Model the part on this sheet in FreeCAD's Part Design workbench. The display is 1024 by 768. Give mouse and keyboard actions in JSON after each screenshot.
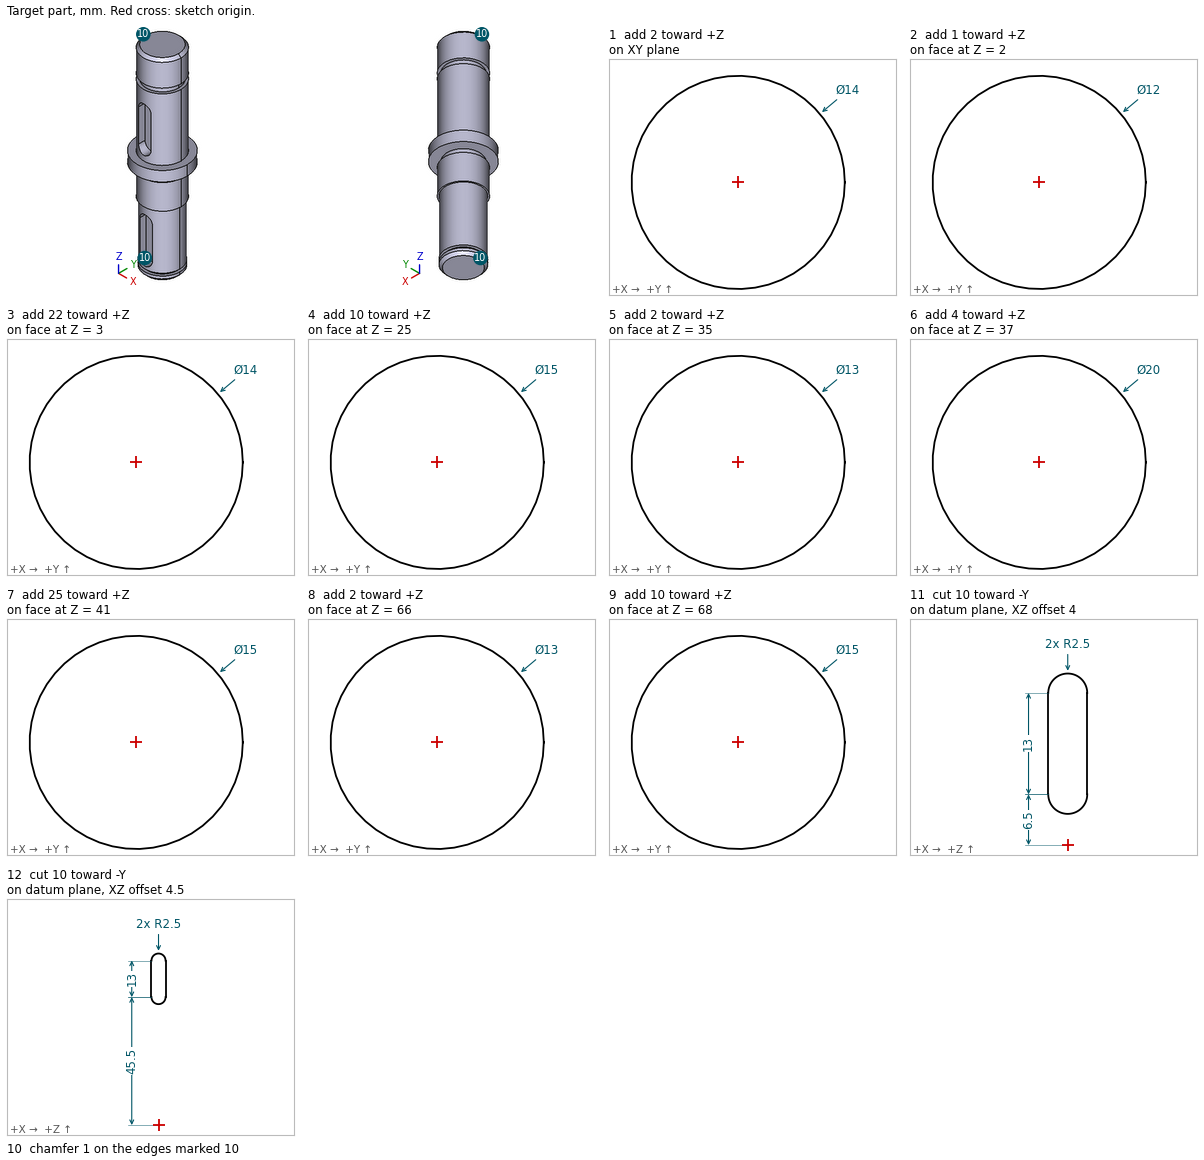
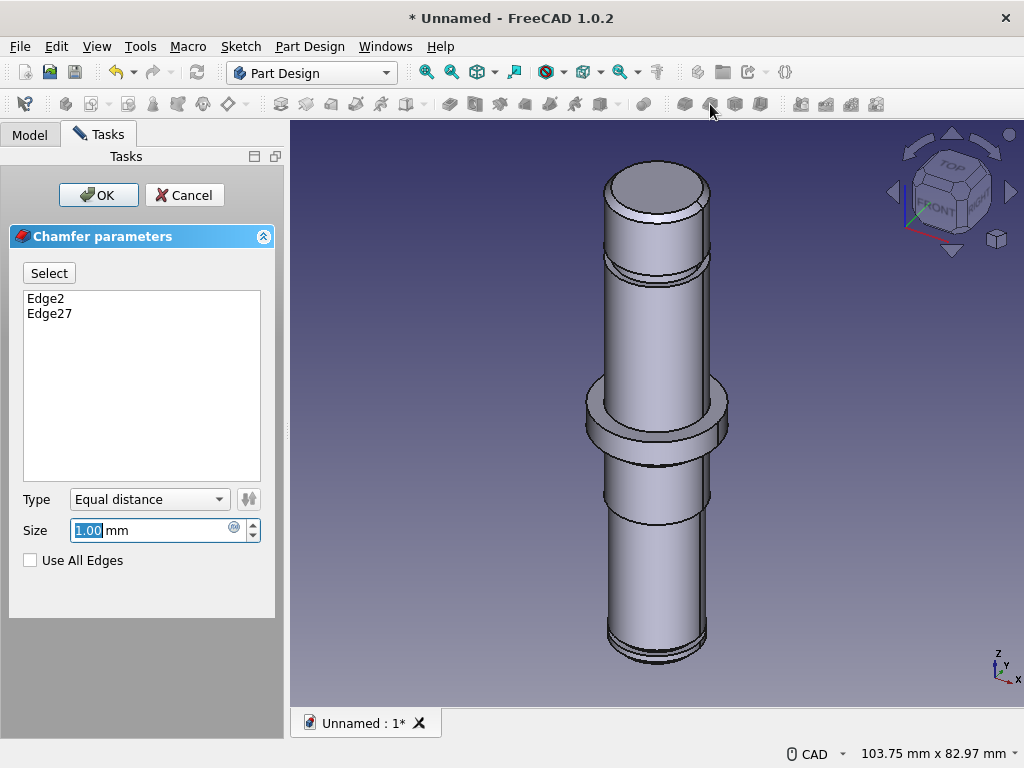
{"action": "type", "text": "1"}
{"action": "key", "text": "Tab"}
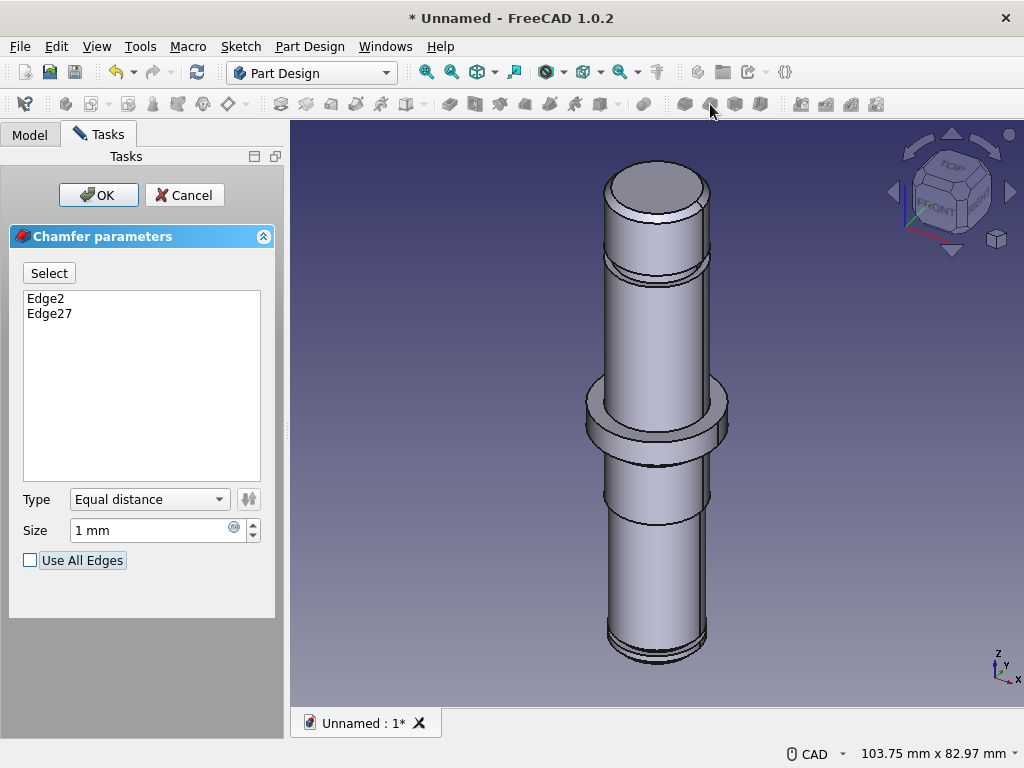
{"action": "left_click", "coordinate": [99, 195]}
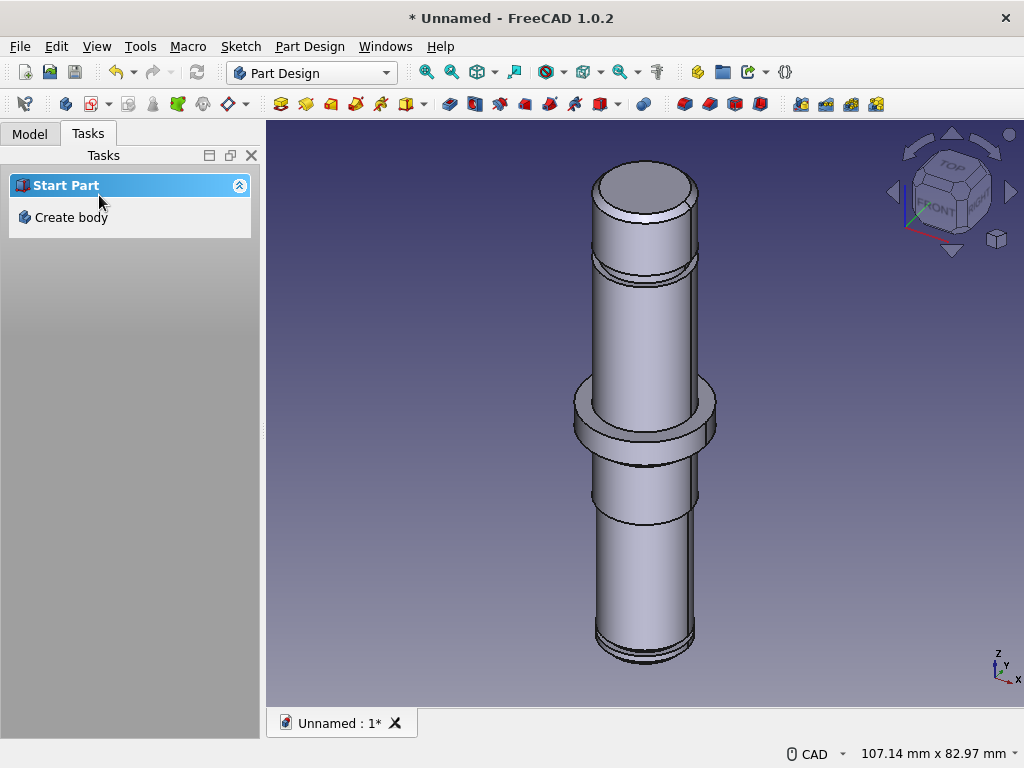
{"action": "left_click", "coordinate": [30, 134]}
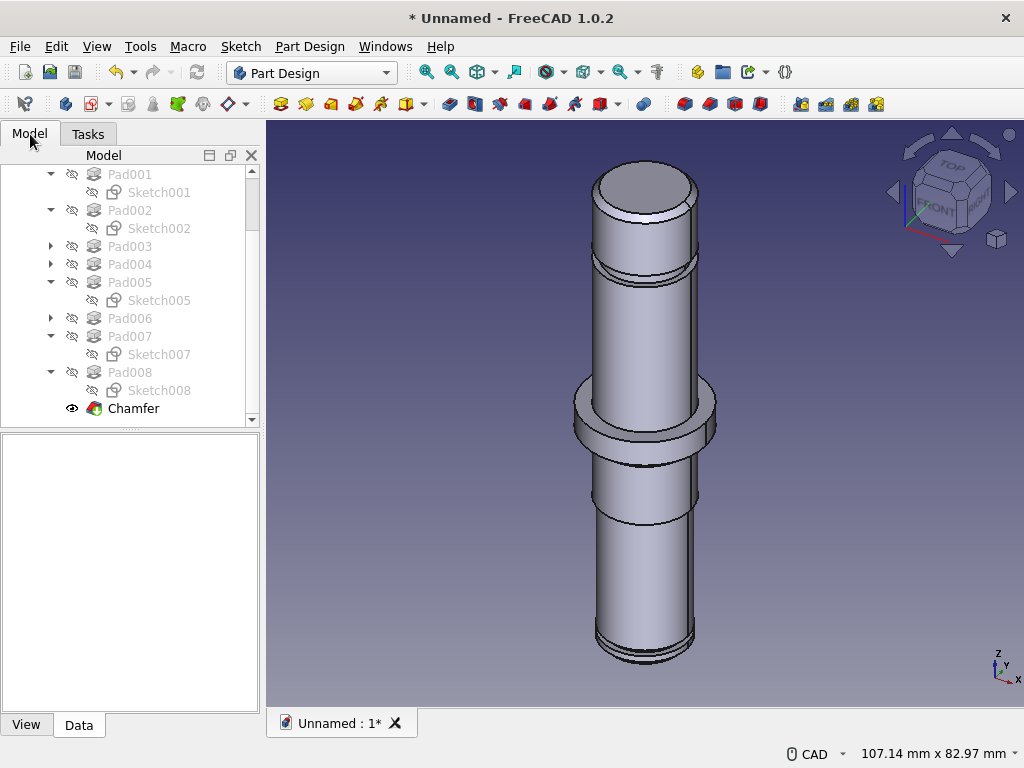
{"action": "scroll", "coordinate": [141, 296], "scroll_direction": "down", "scroll_amount": 3}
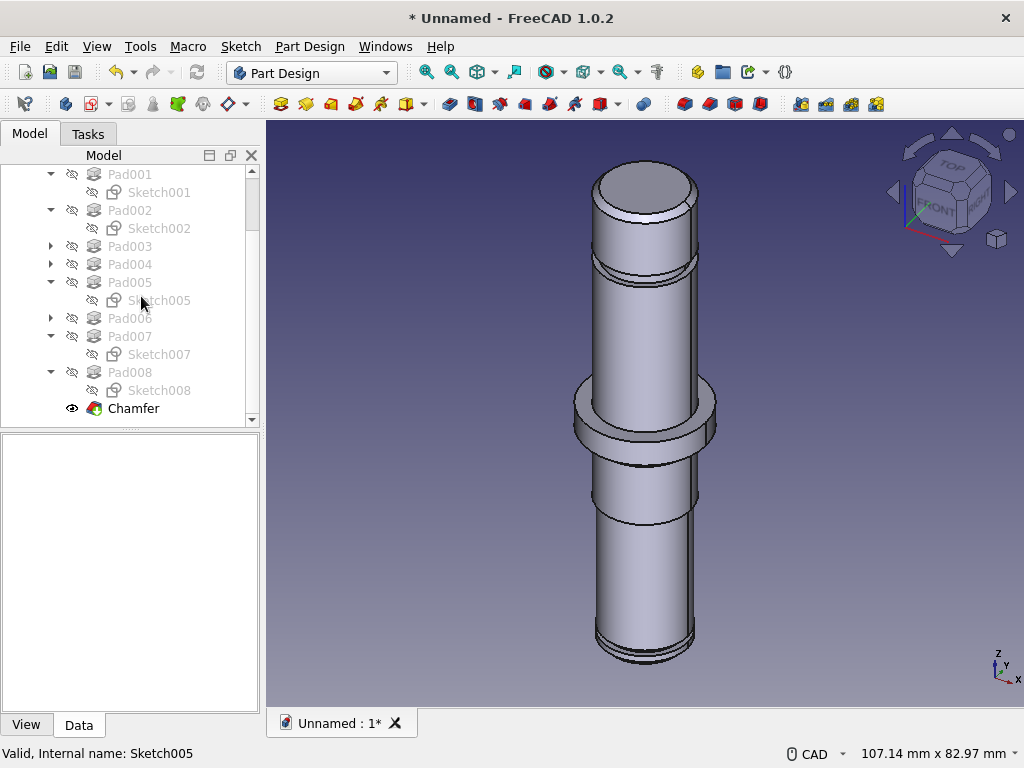
{"action": "scroll", "coordinate": [141, 296], "scroll_direction": "up", "scroll_amount": 15}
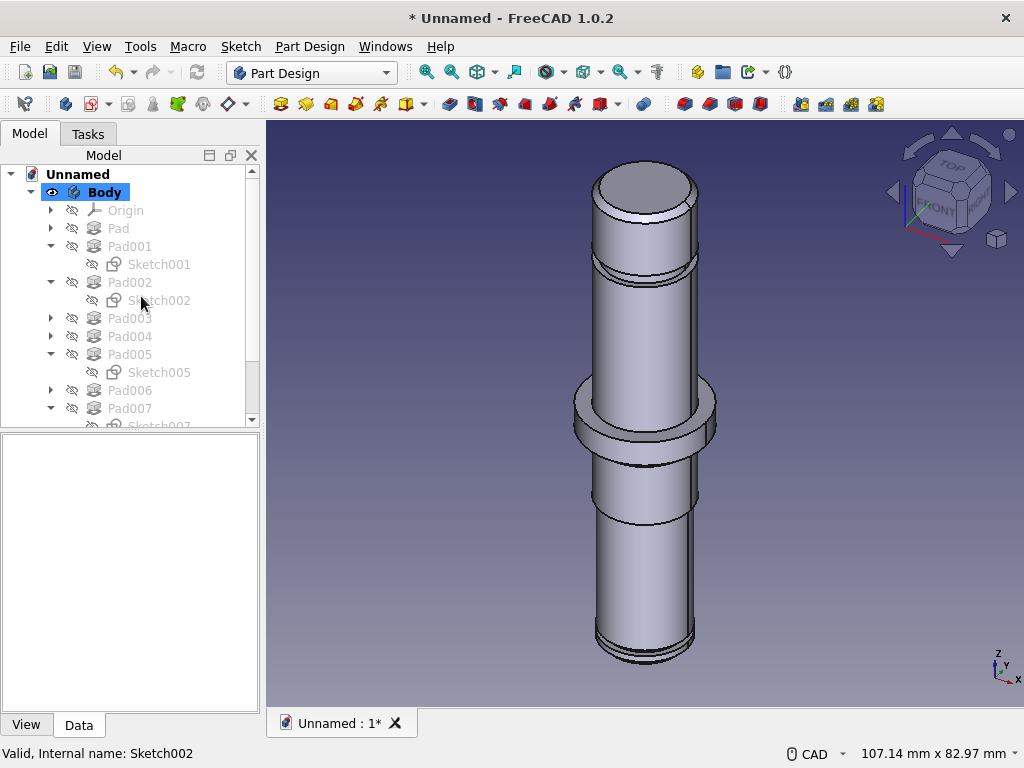
{"action": "left_click", "coordinate": [51, 210]}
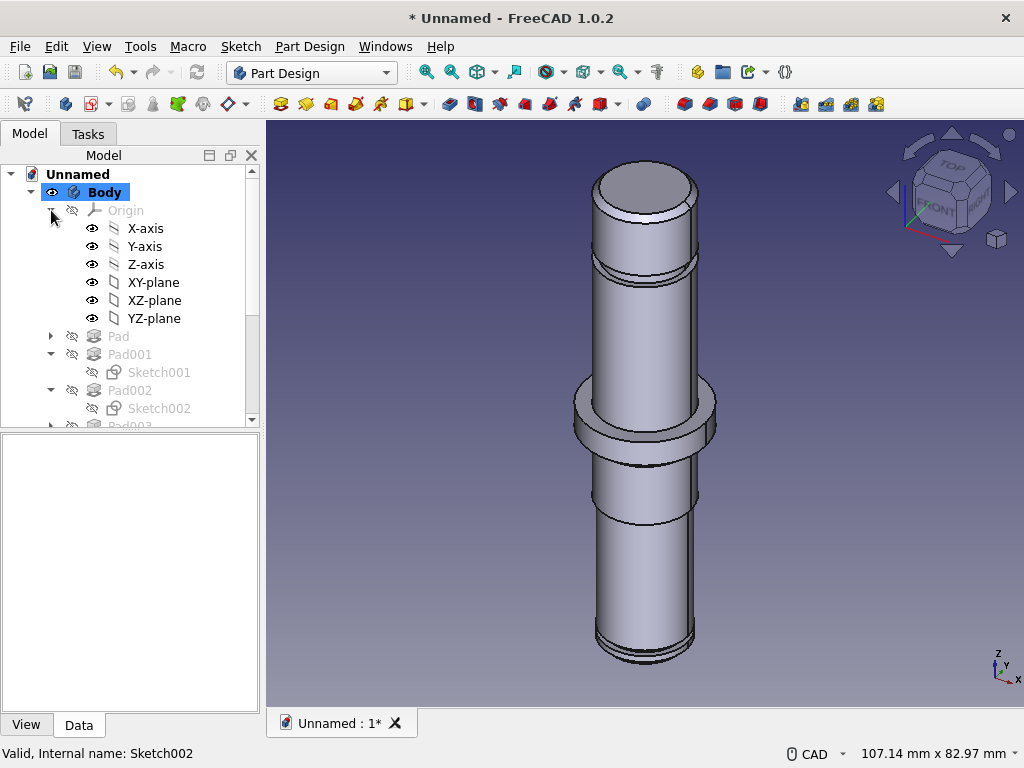
{"action": "left_click", "coordinate": [137, 300]}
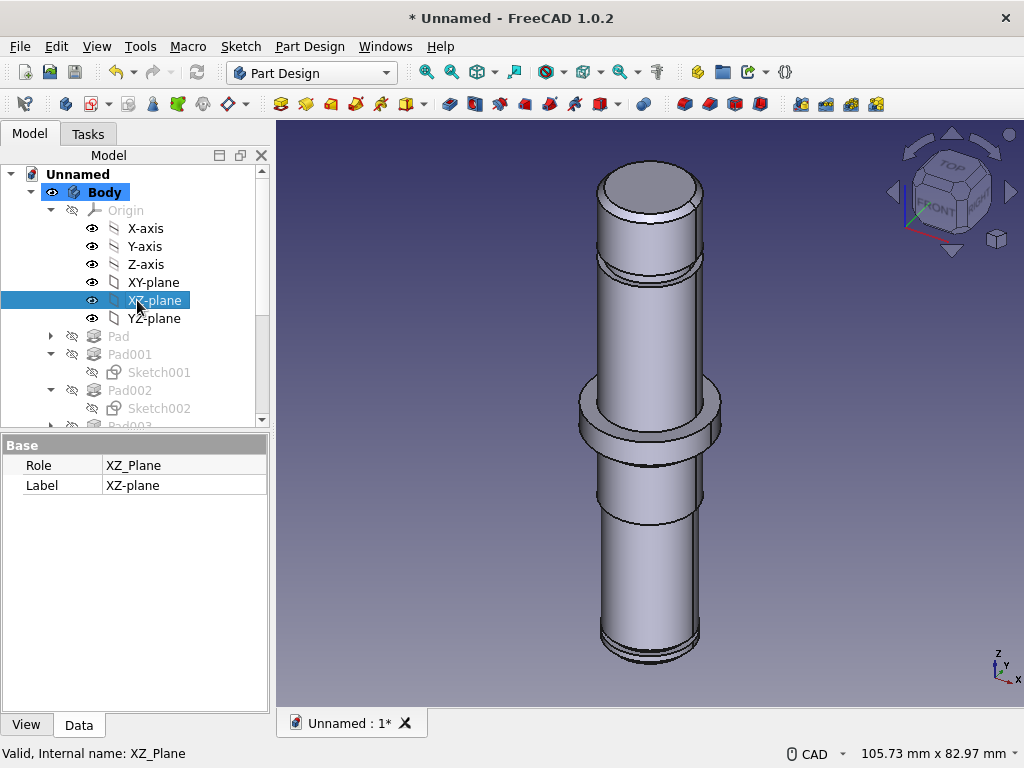
{"action": "left_click", "coordinate": [228, 104]}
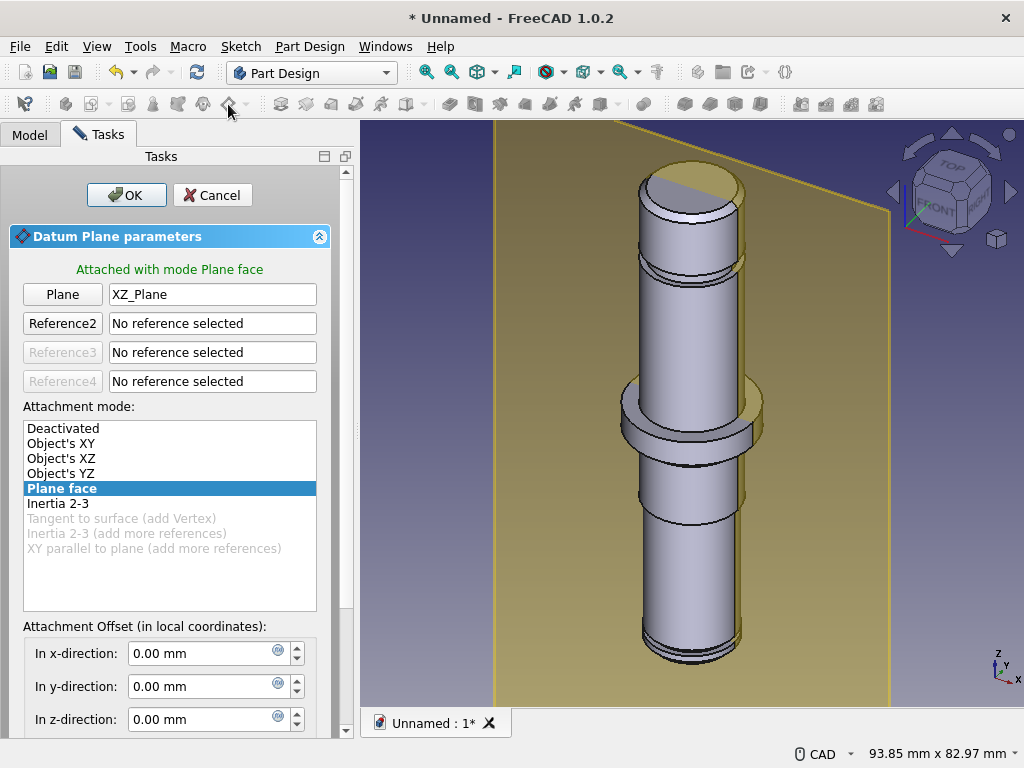
{"action": "triple_click", "coordinate": [210, 720]}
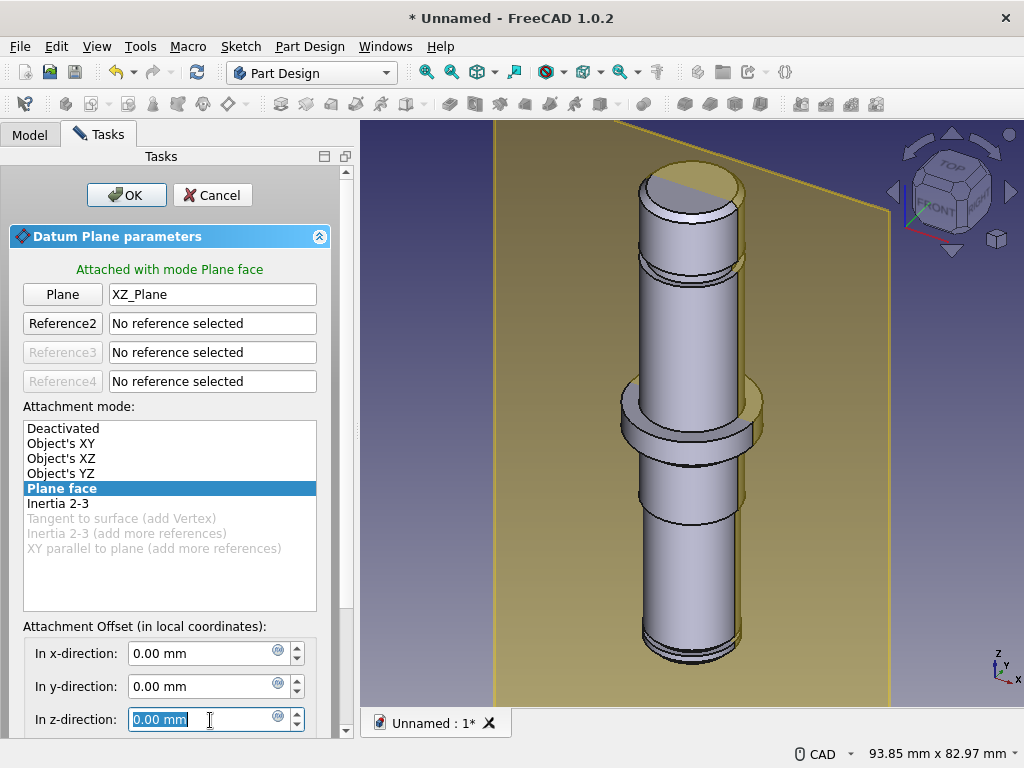
{"action": "type", "text": "4"}
{"action": "key", "text": "Tab"}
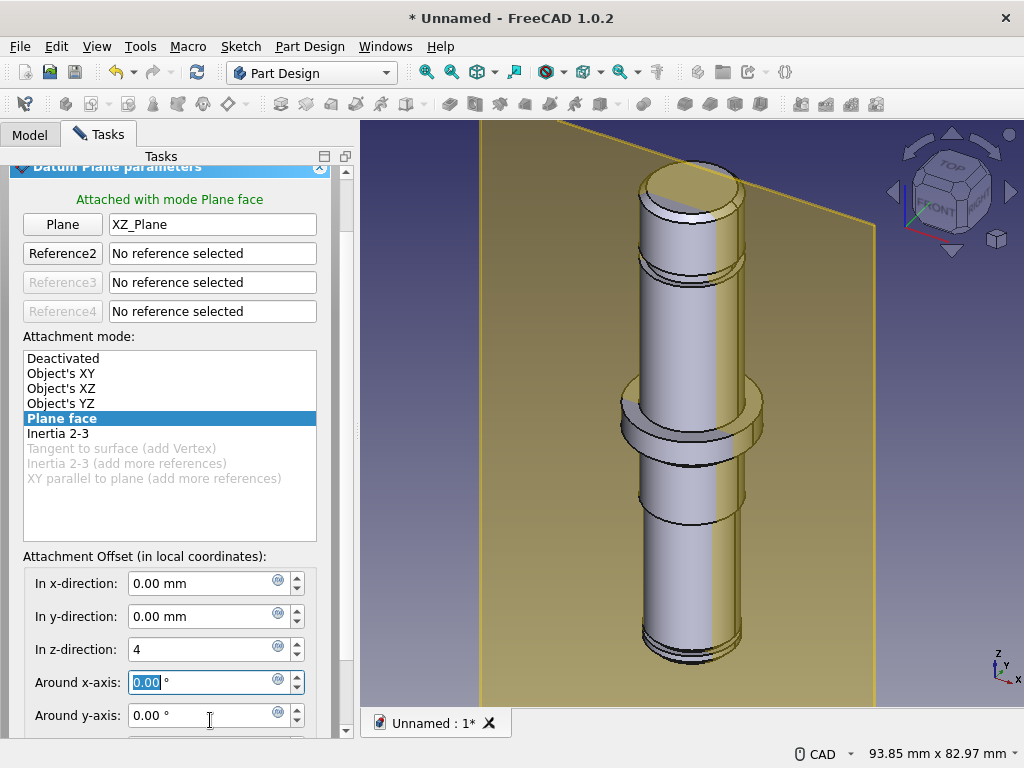
{"action": "scroll", "coordinate": [346, 452], "scroll_direction": "up", "scroll_amount": 2}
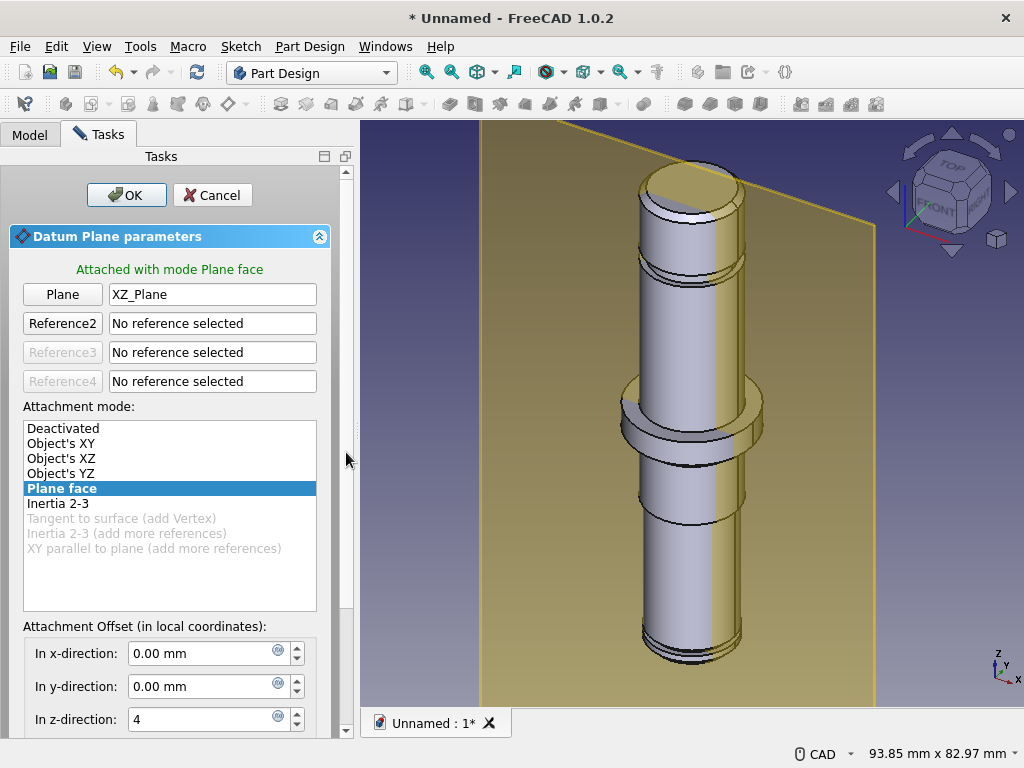
{"action": "left_click", "coordinate": [127, 195]}